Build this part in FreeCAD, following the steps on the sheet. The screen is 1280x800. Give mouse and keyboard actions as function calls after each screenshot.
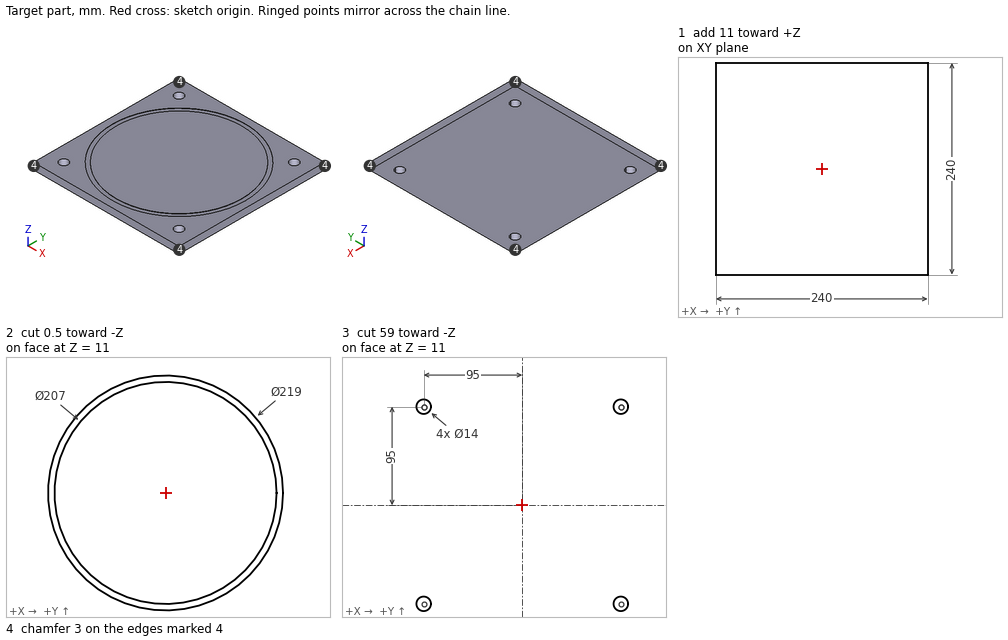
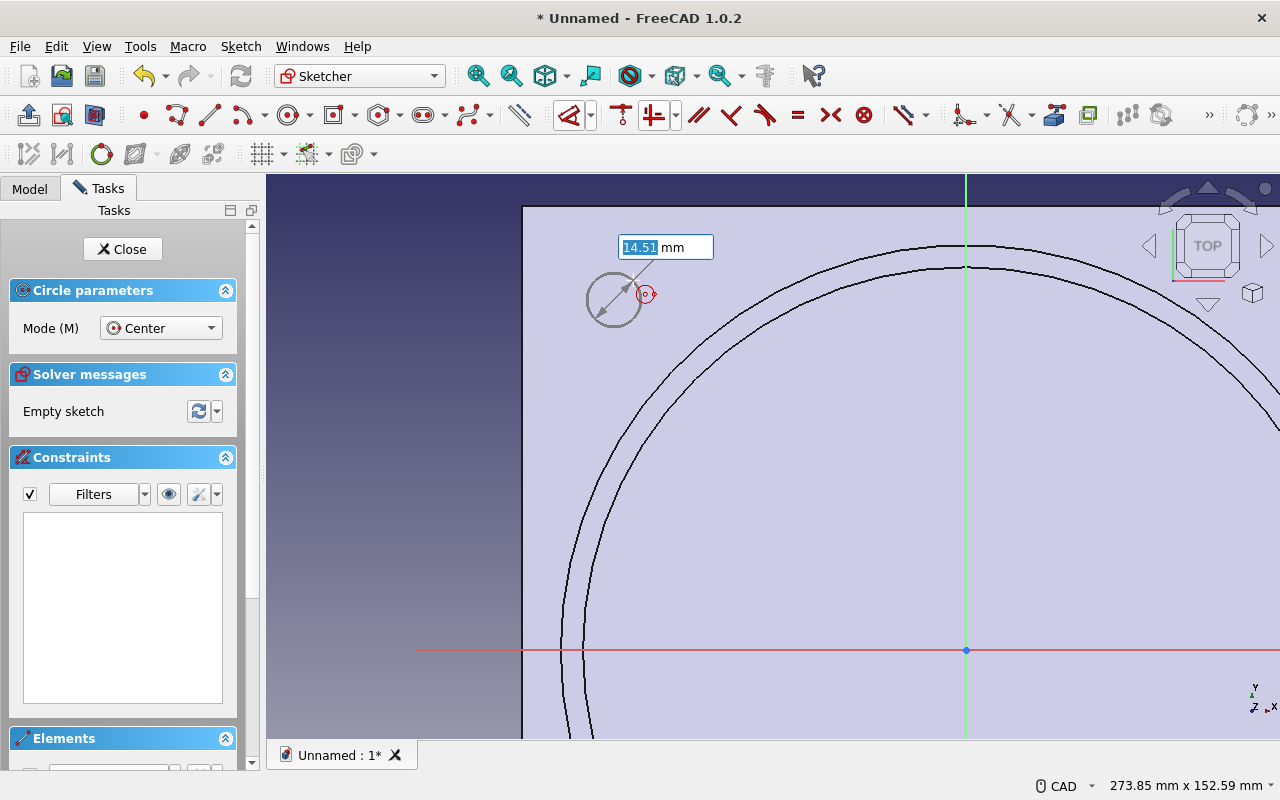
text(14)
key(Return)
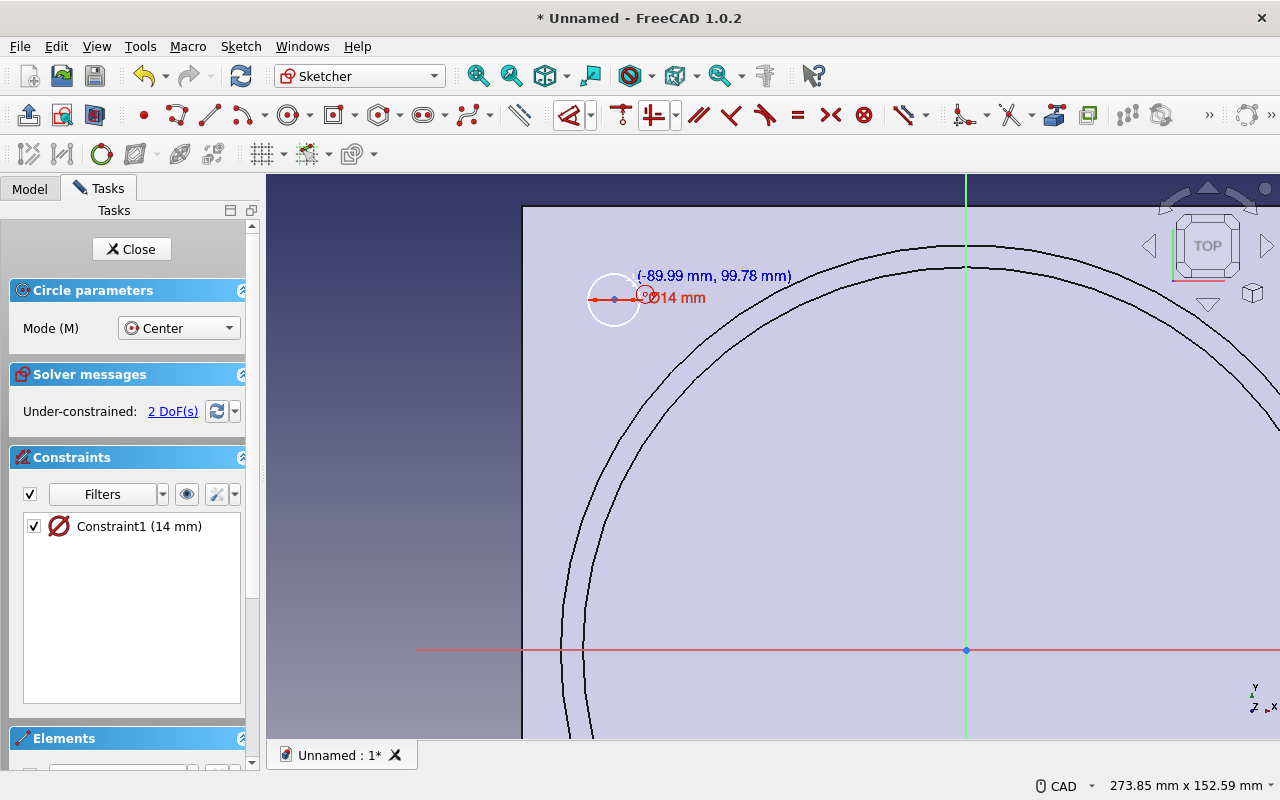
scroll(491, 298, down, 4)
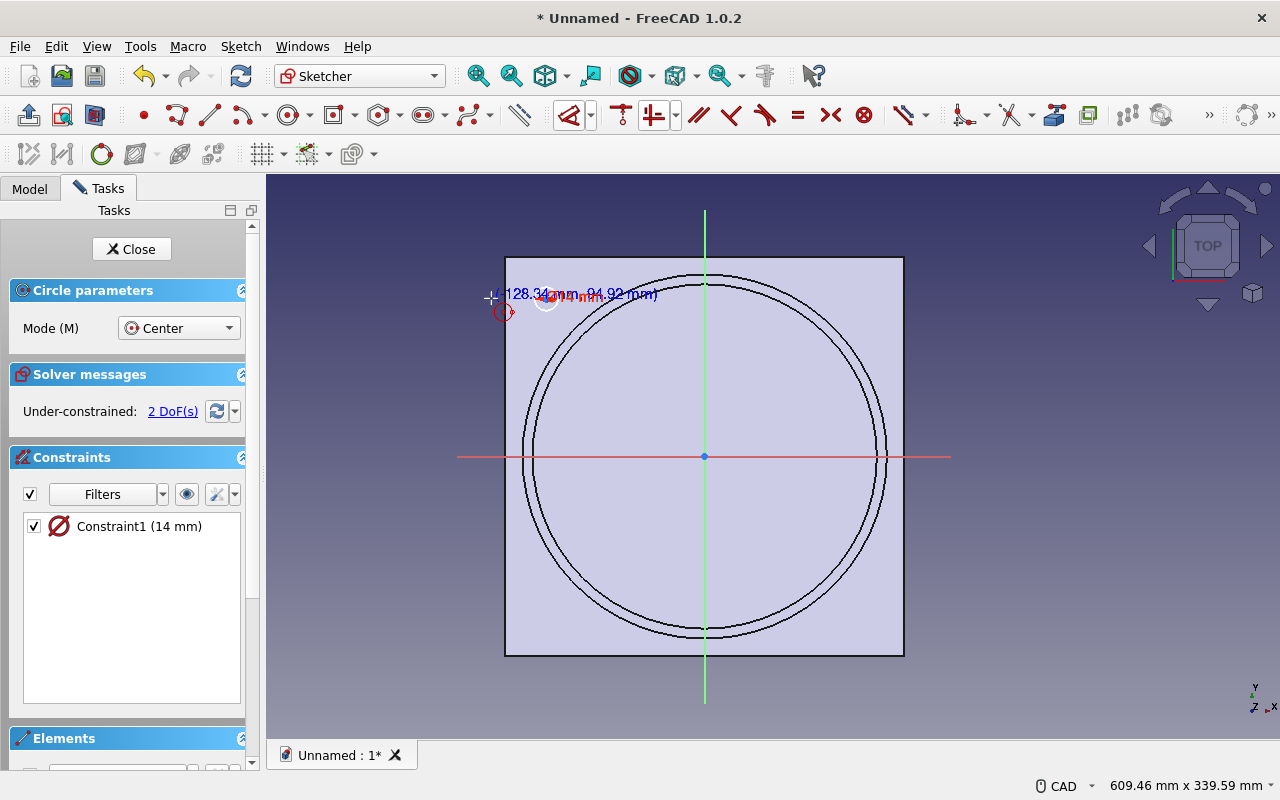
scroll(863, 298, up, 4)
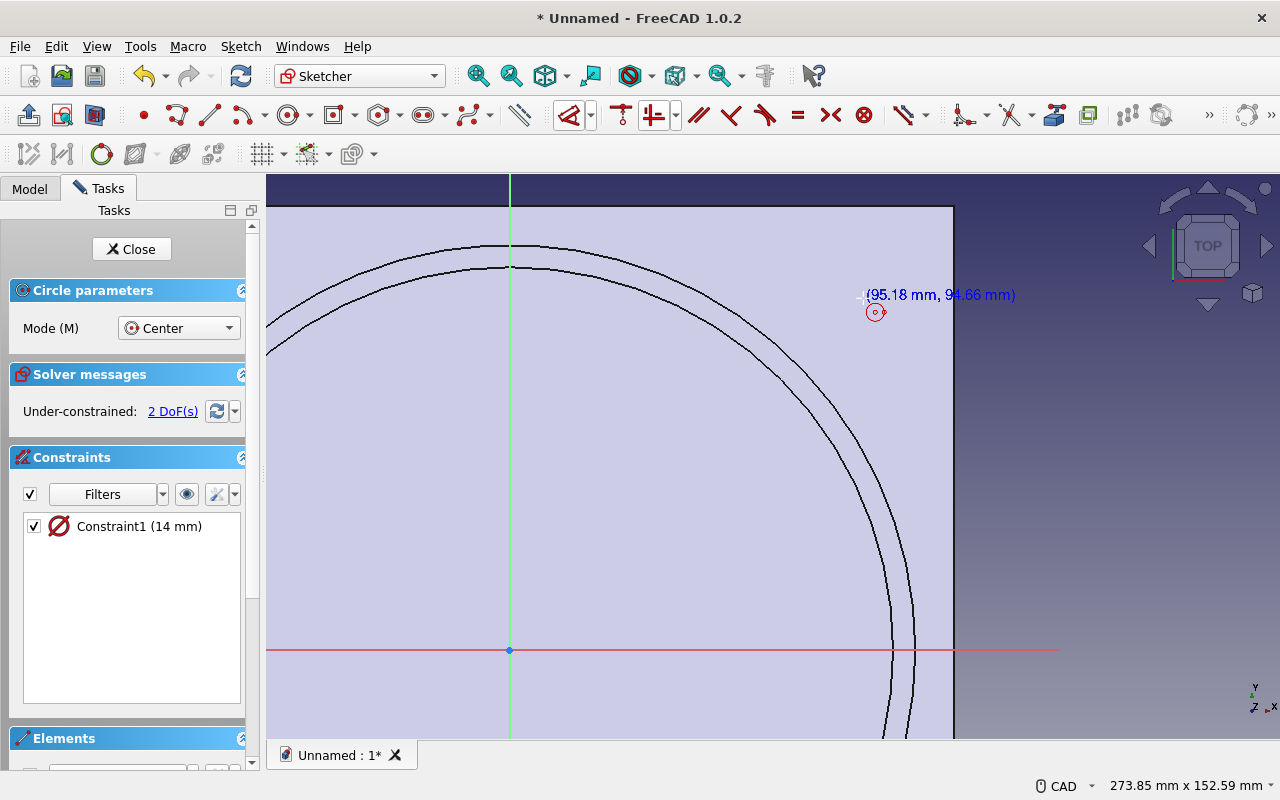
click(862, 299)
move(880, 280)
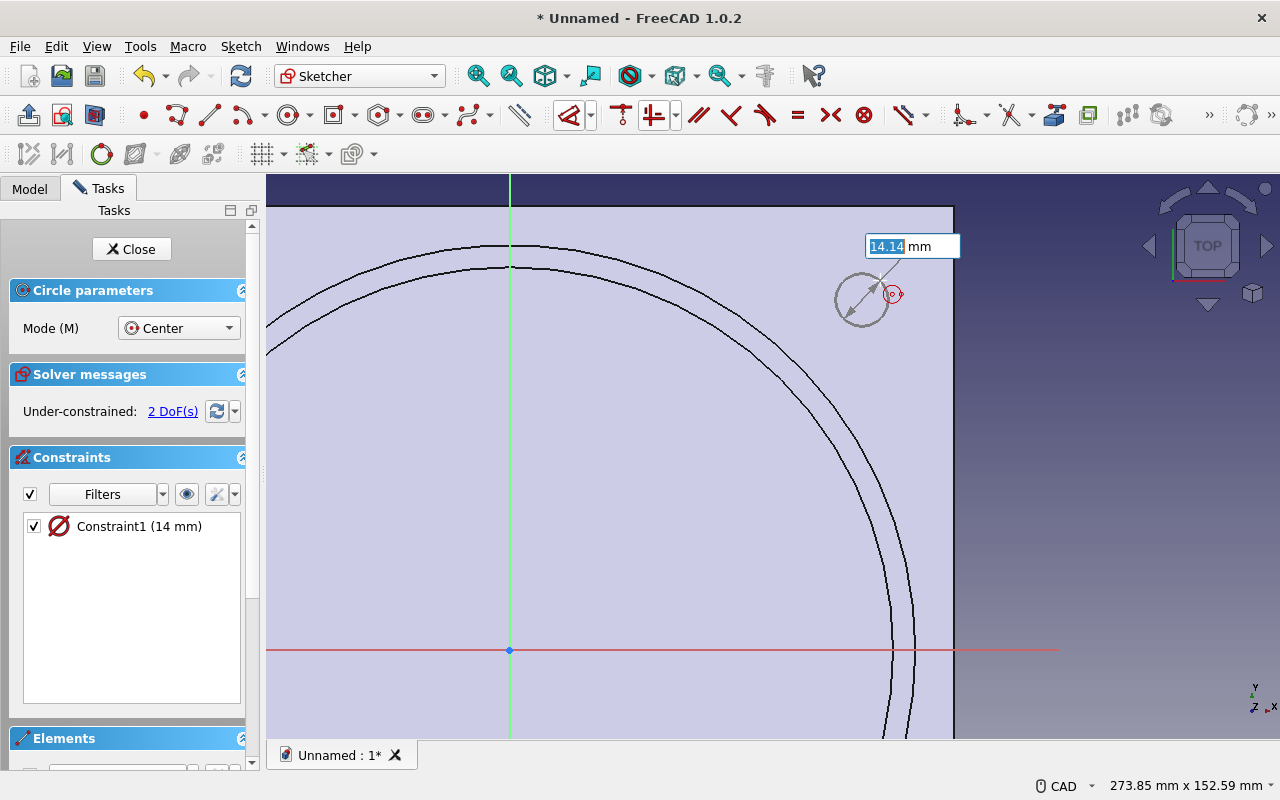
text(14)
key(Return)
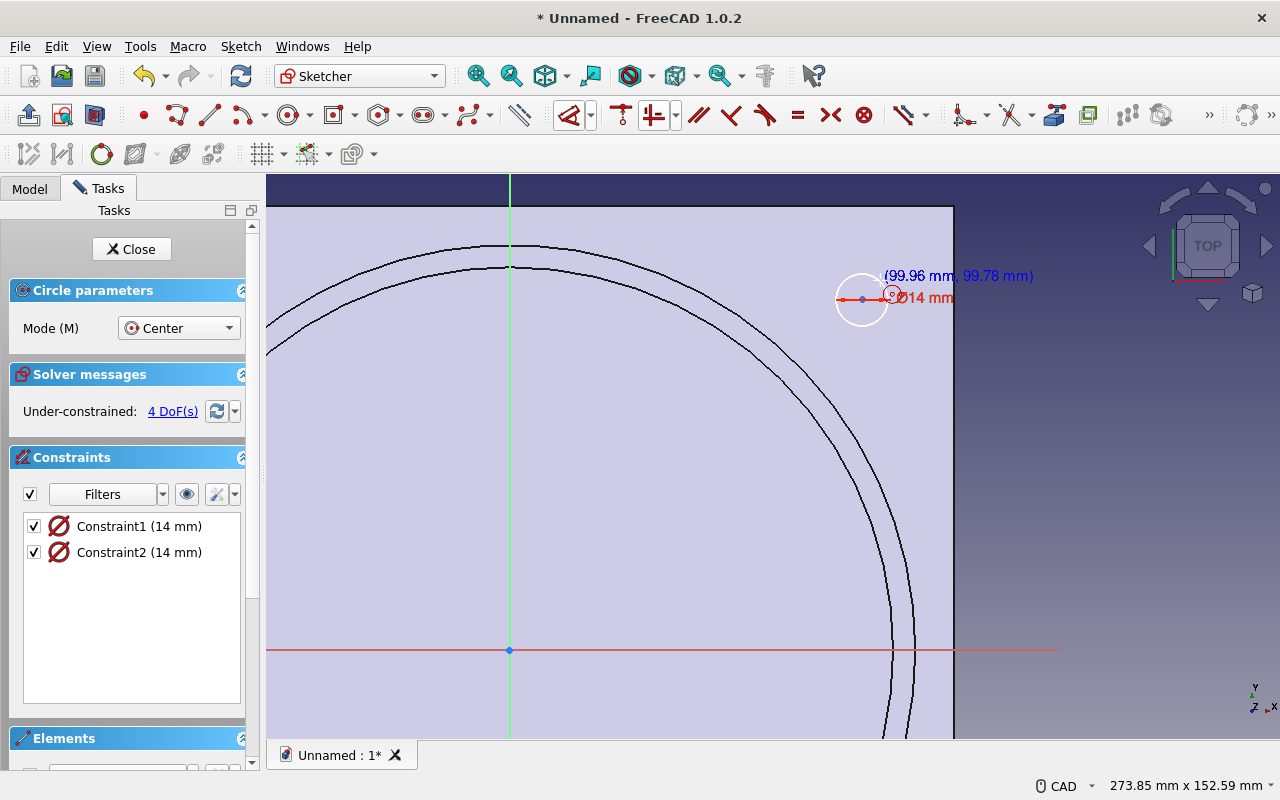
scroll(863, 298, down, 4)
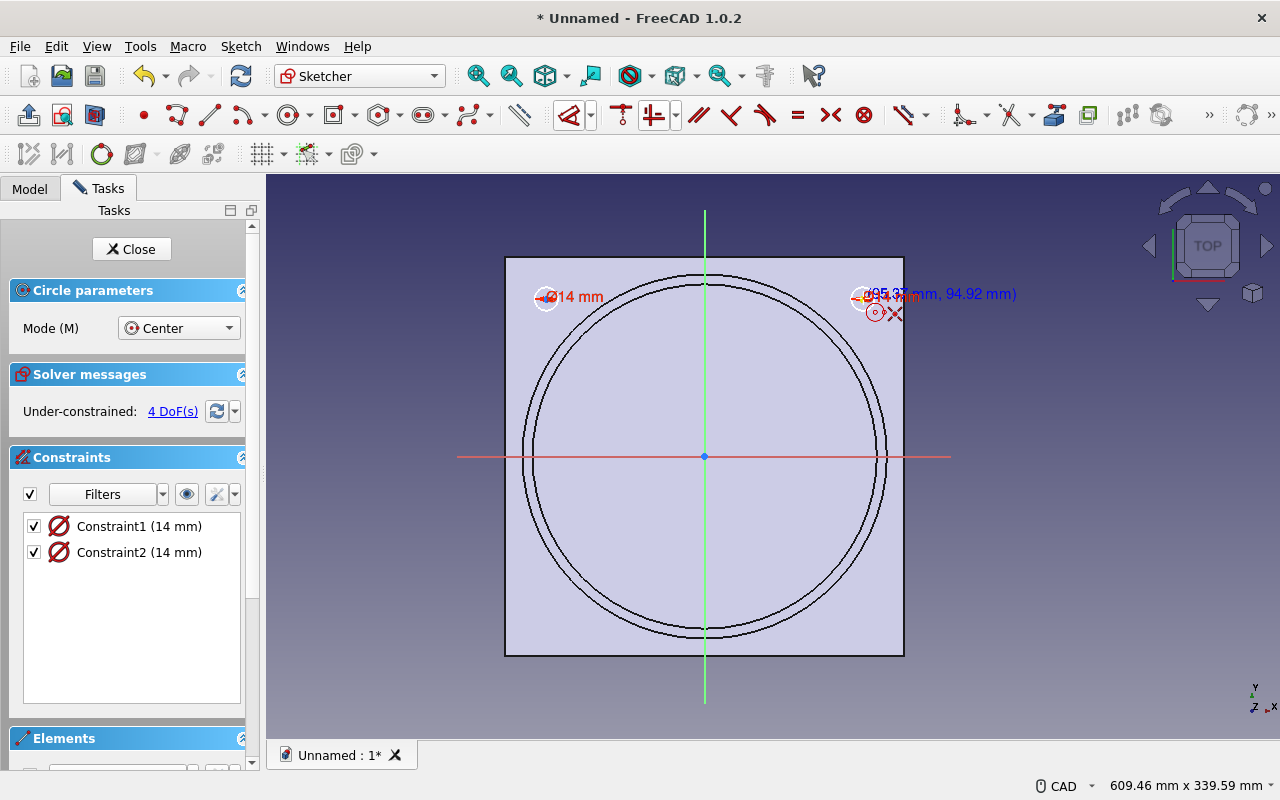
scroll(863, 615, up, 4)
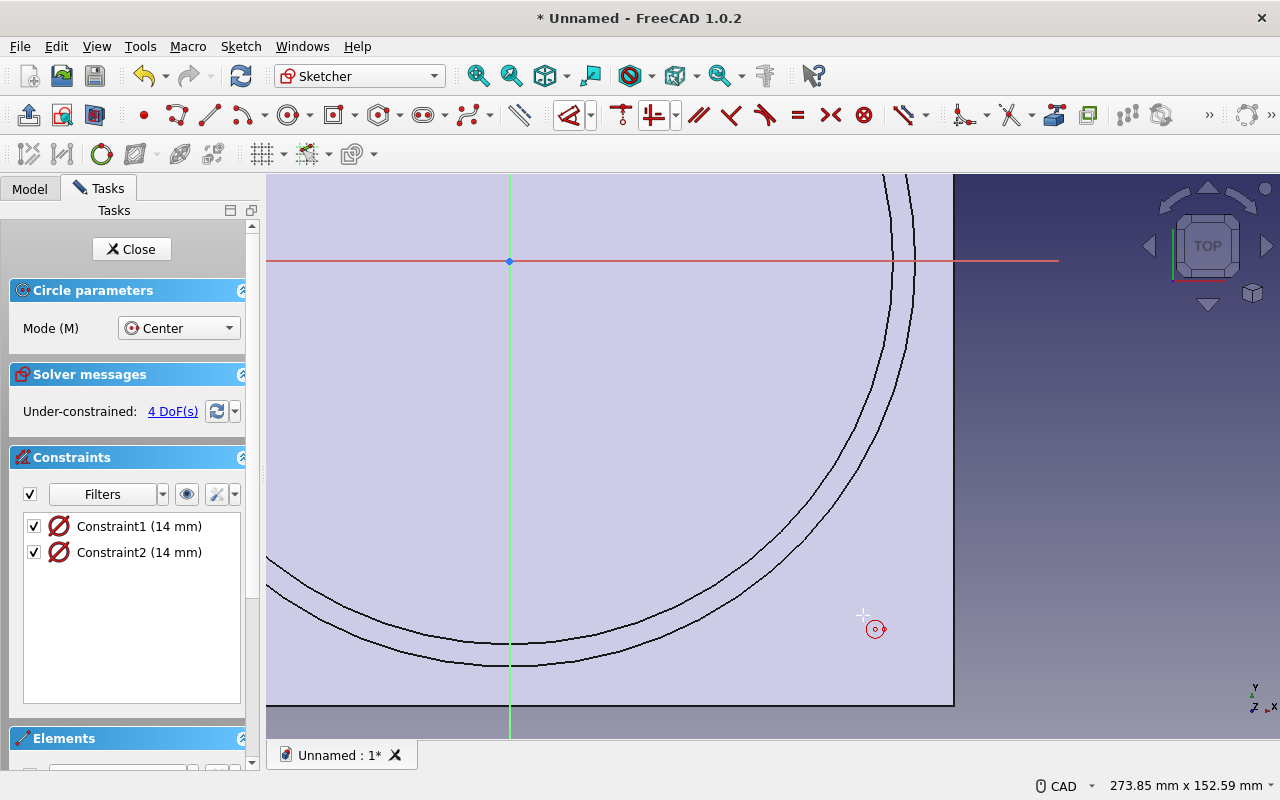
click(862, 613)
move(880, 595)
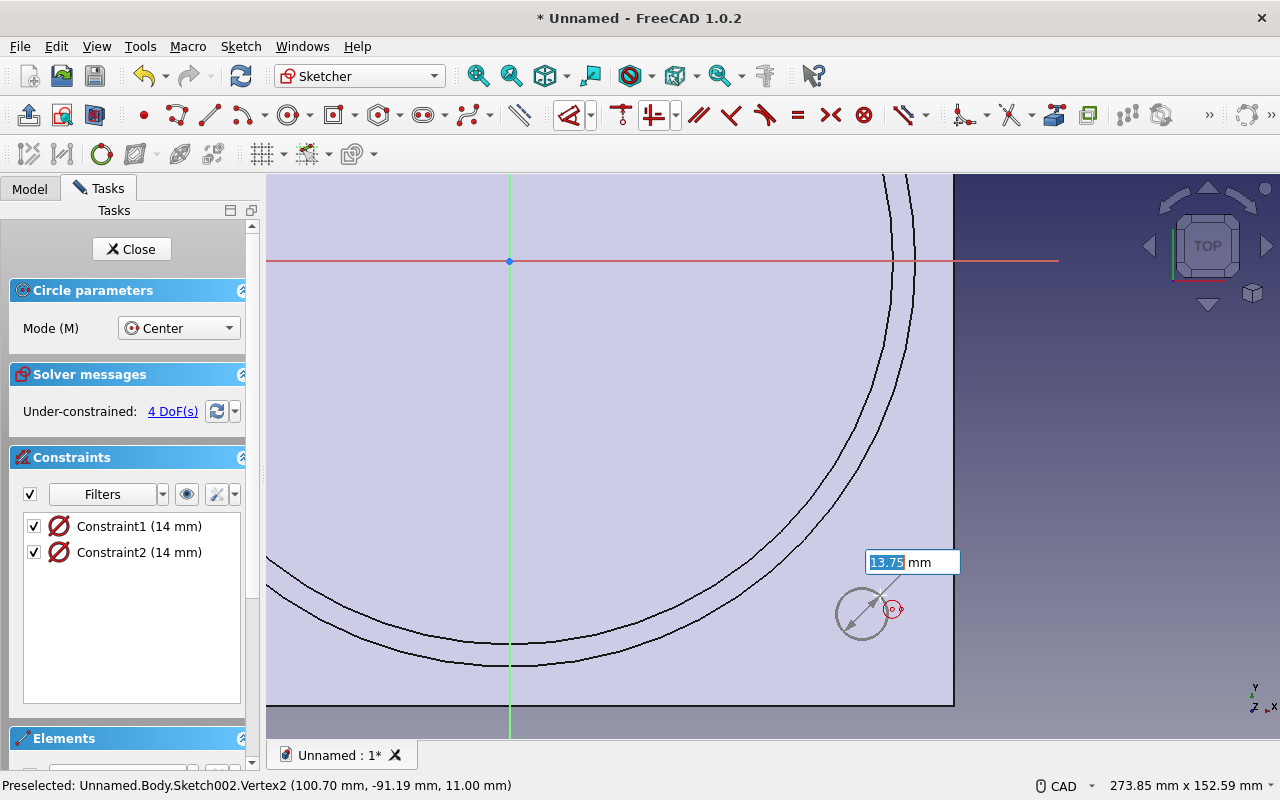
text(14)
key(Return)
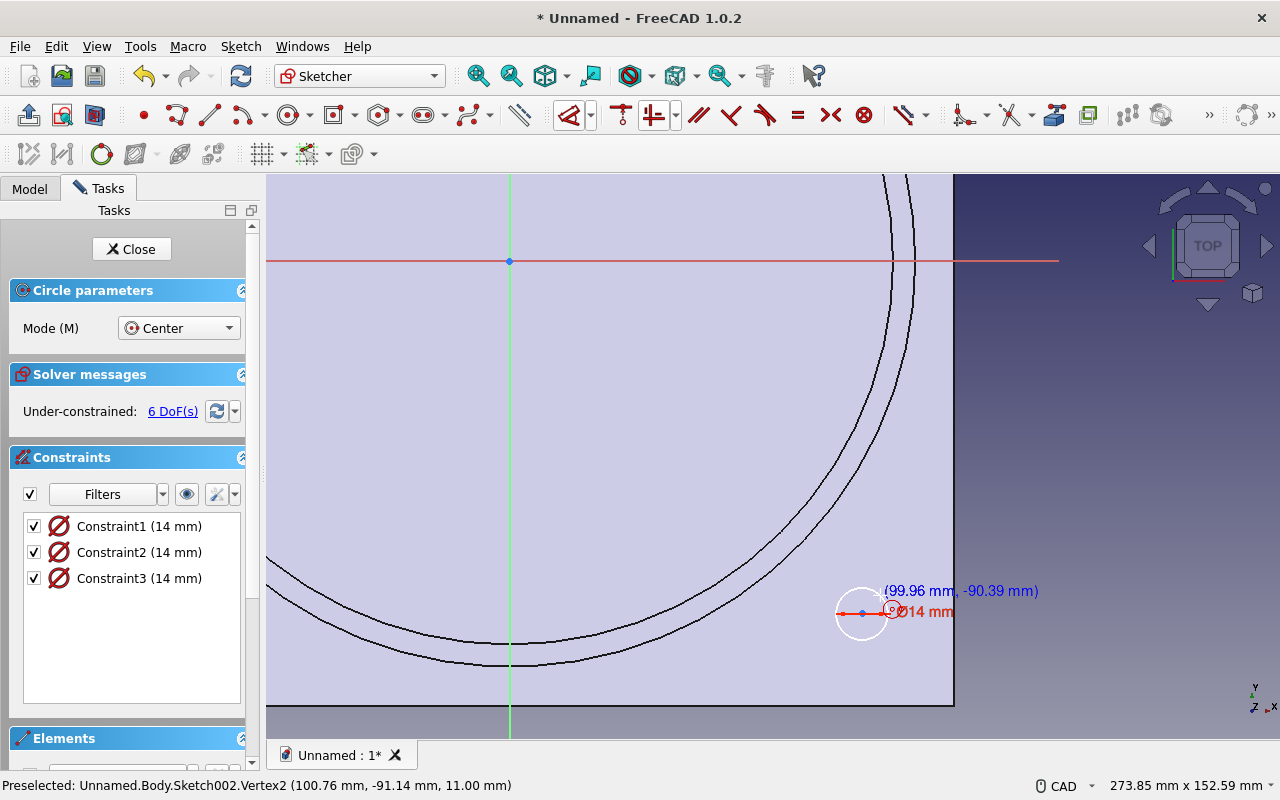
scroll(863, 616, down, 4)